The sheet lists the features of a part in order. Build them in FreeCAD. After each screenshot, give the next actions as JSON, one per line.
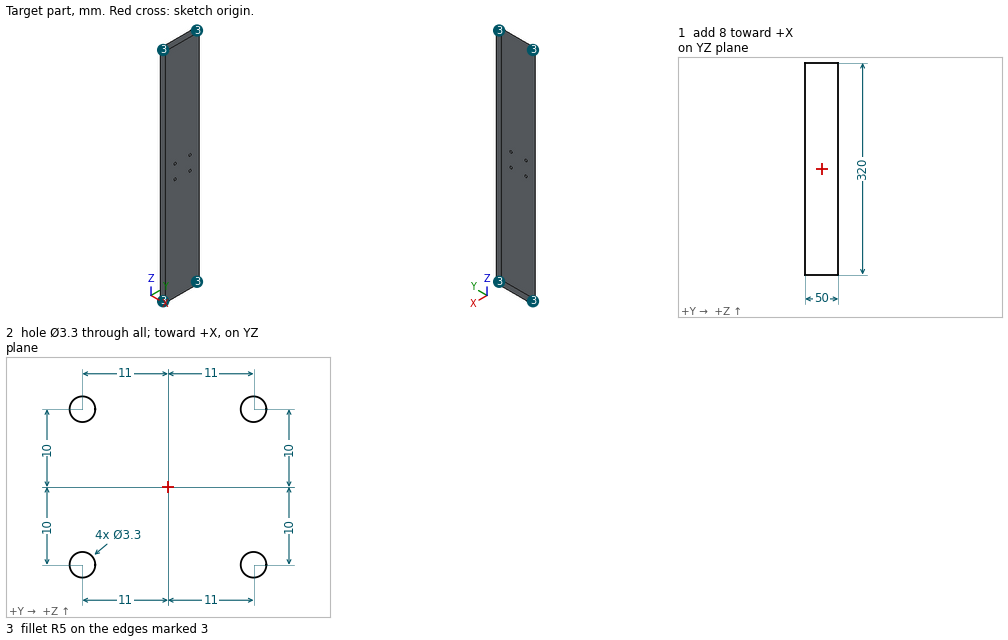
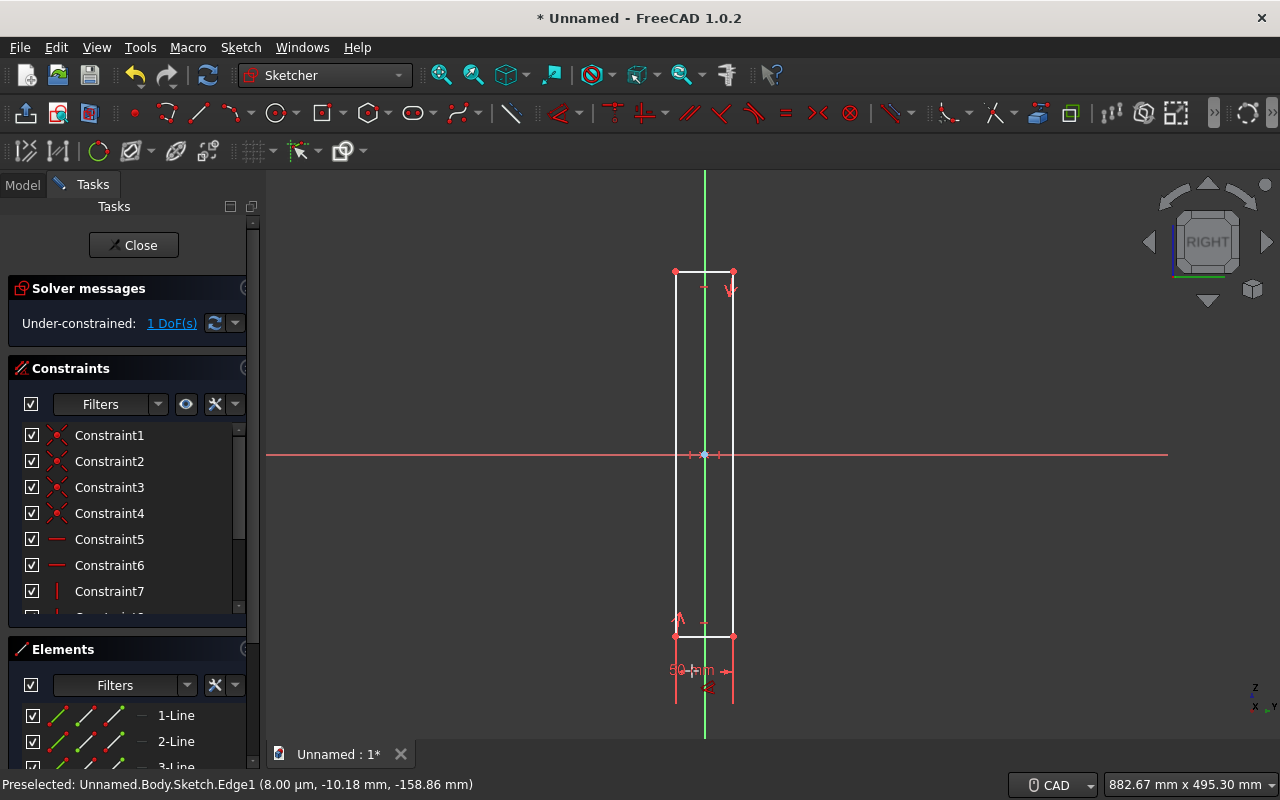
{"action": "left_click", "coordinate": [733, 528]}
{"action": "left_click", "coordinate": [767, 371]}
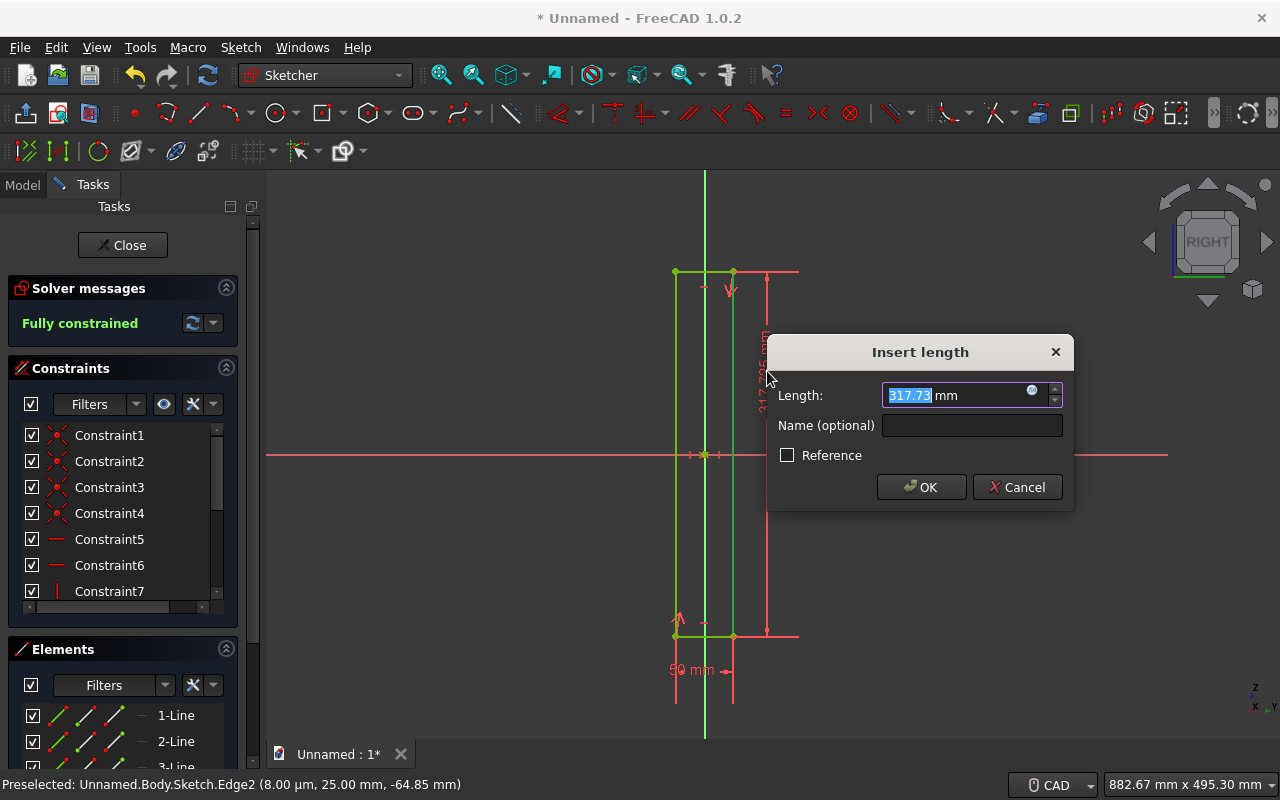
{"action": "type", "text": "320"}
{"action": "key", "text": "Return"}
{"action": "key", "text": "Escape"}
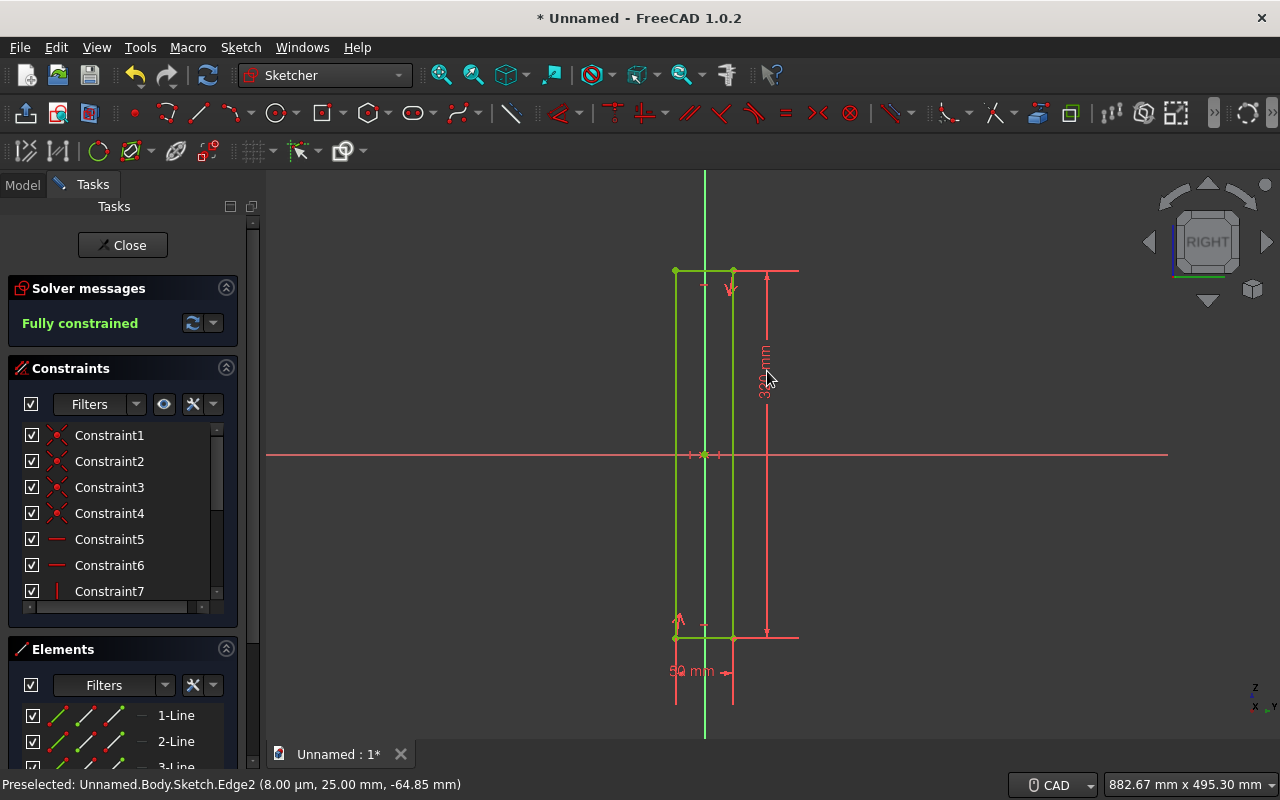
{"action": "left_click", "coordinate": [123, 245]}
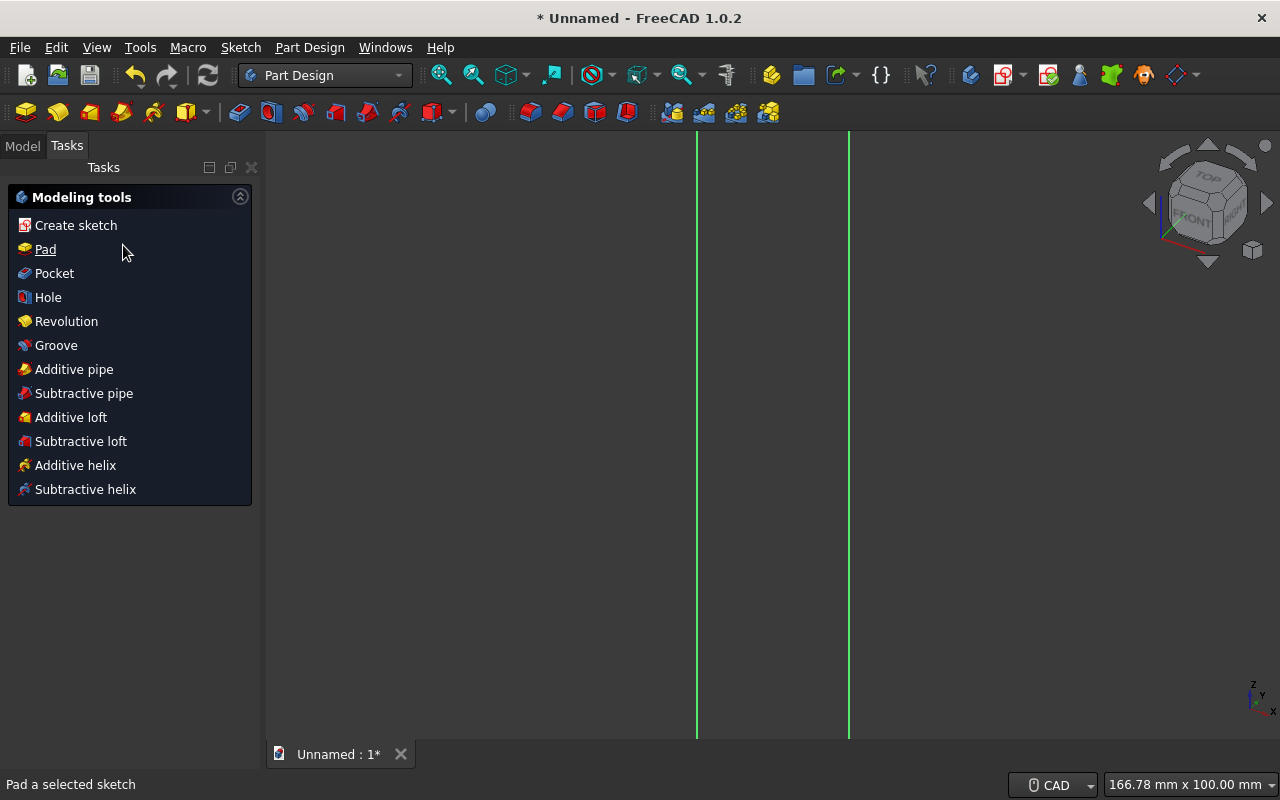
{"action": "left_click", "coordinate": [26, 112]}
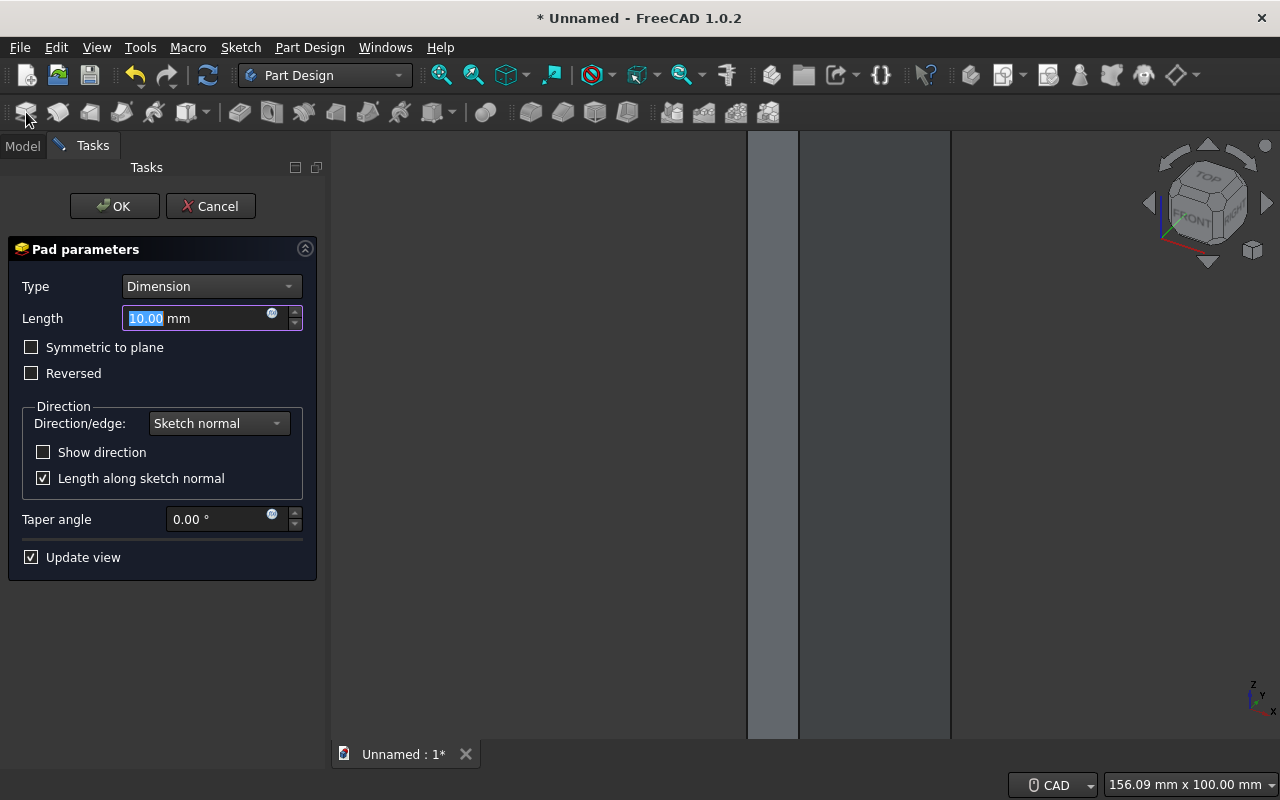
{"action": "type", "text": "8"}
{"action": "key", "text": "Tab"}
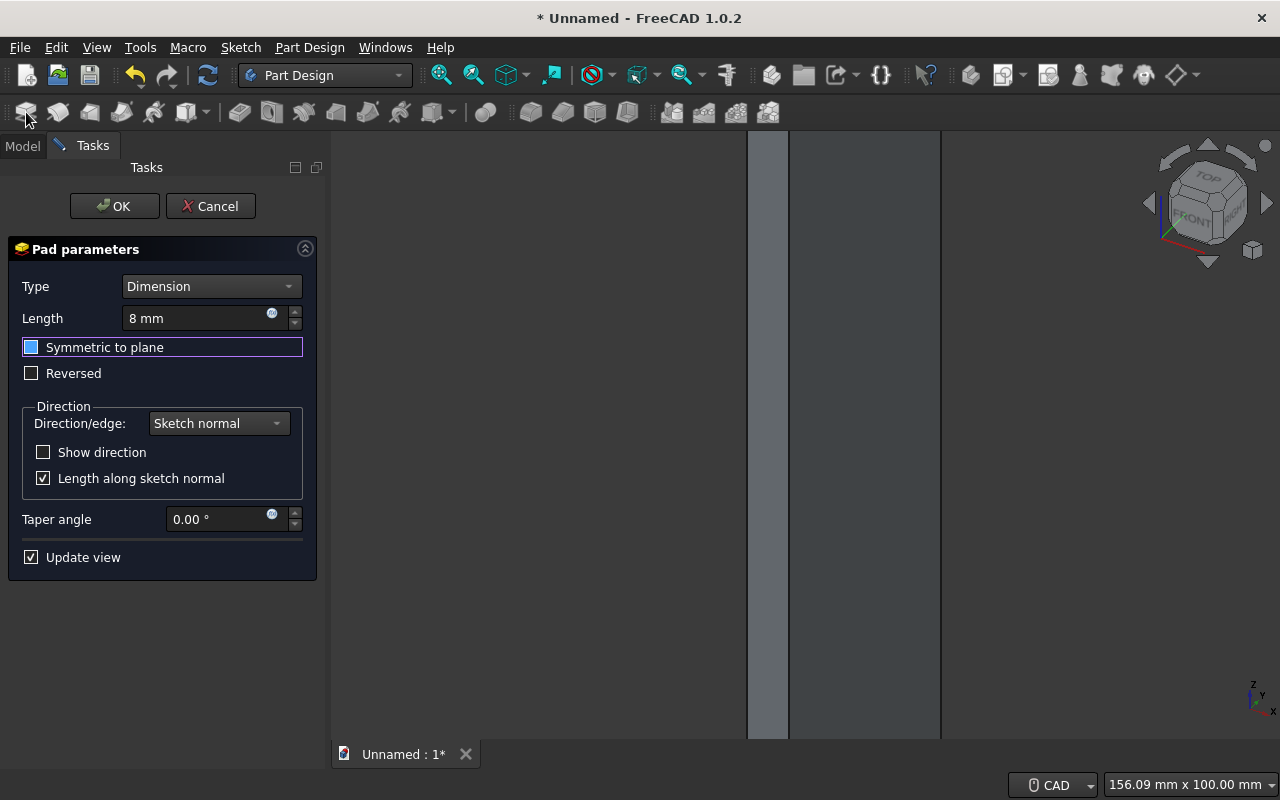
{"action": "left_click", "coordinate": [115, 206]}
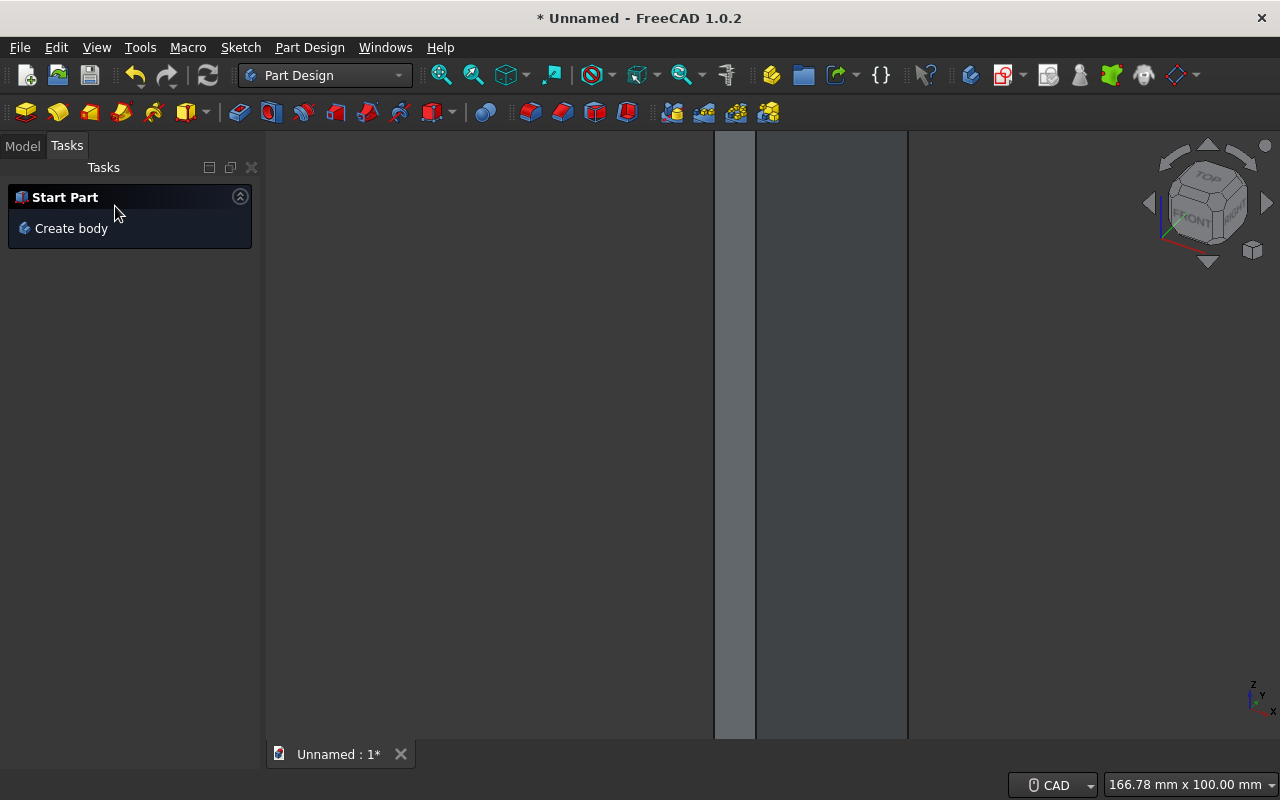
{"action": "left_click", "coordinate": [442, 76]}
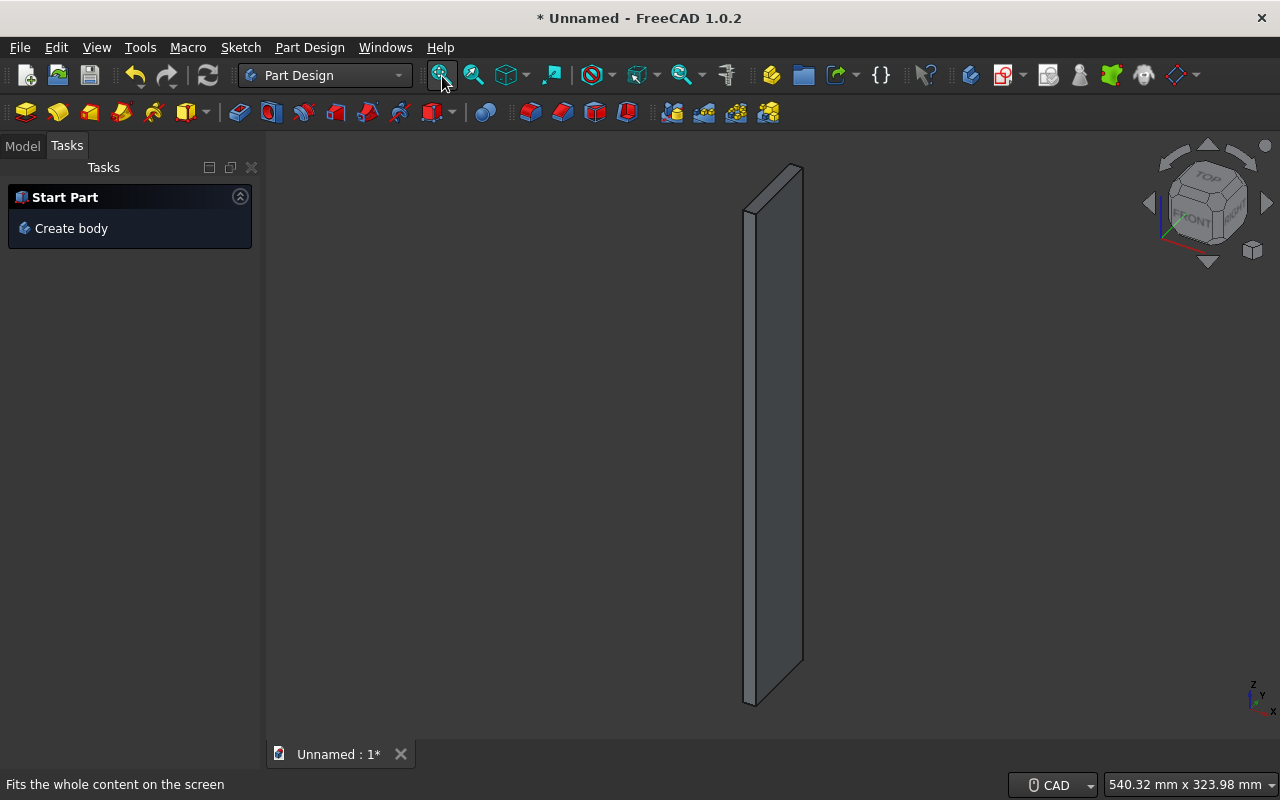
{"action": "left_click", "coordinate": [1004, 76]}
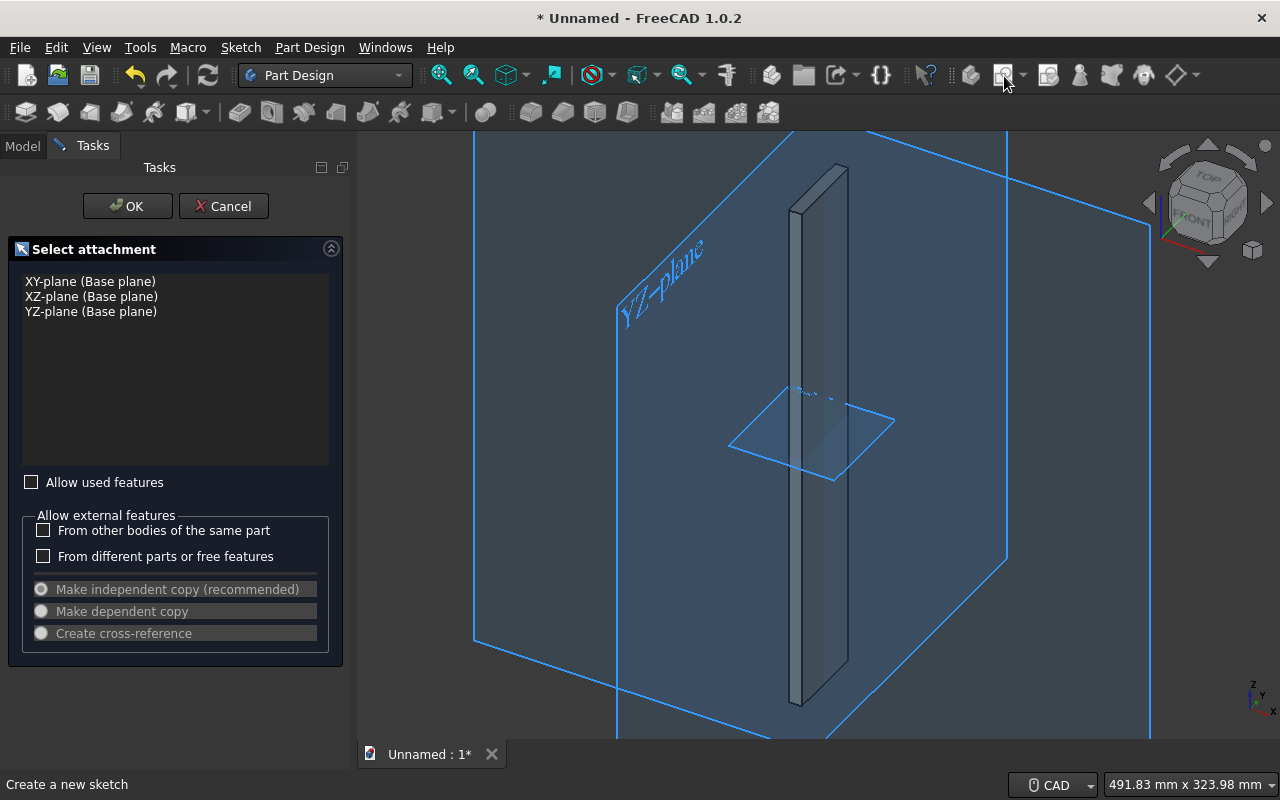
{"action": "left_click", "coordinate": [82, 312]}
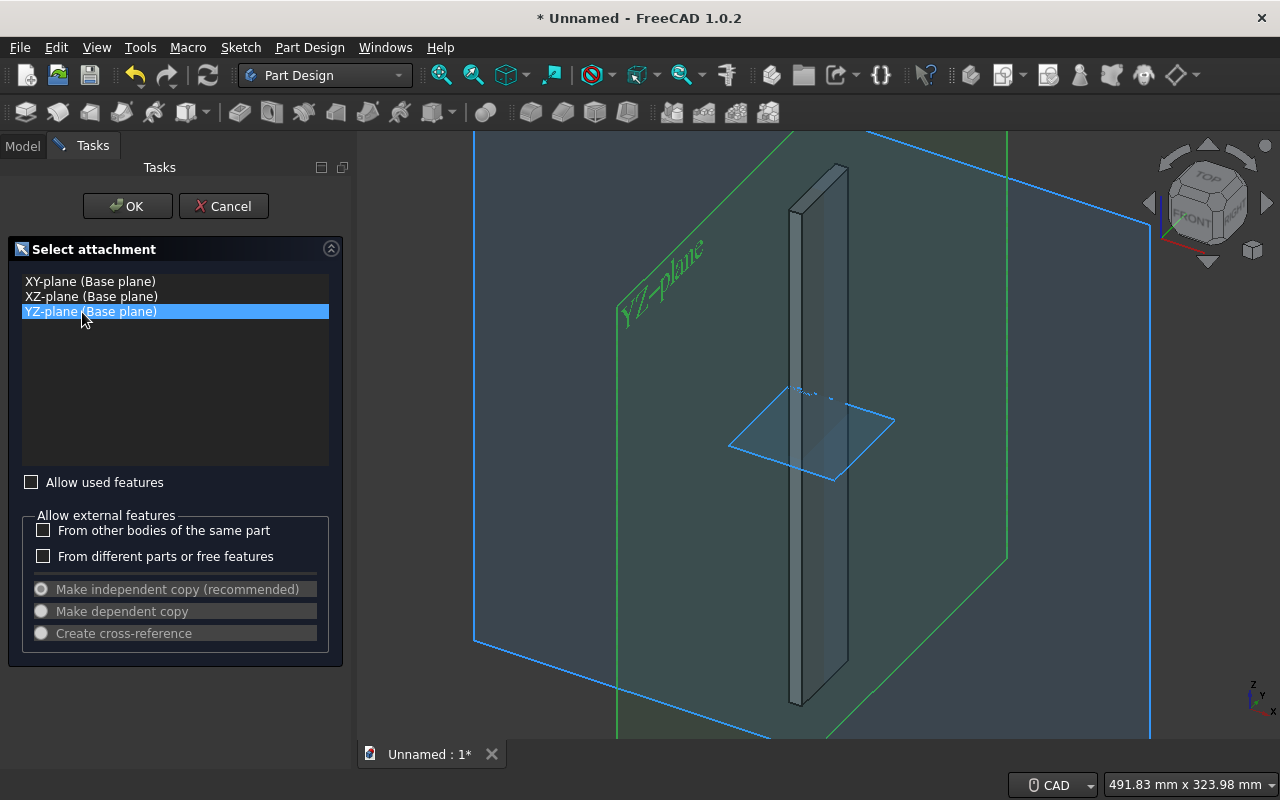
{"action": "left_click", "coordinate": [128, 206]}